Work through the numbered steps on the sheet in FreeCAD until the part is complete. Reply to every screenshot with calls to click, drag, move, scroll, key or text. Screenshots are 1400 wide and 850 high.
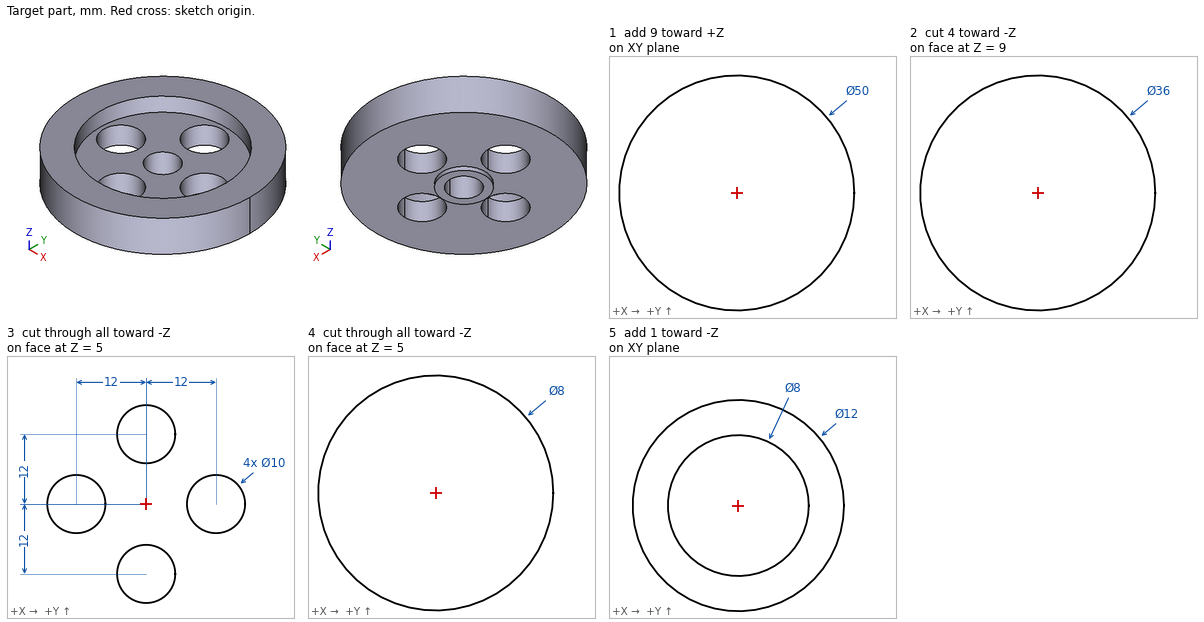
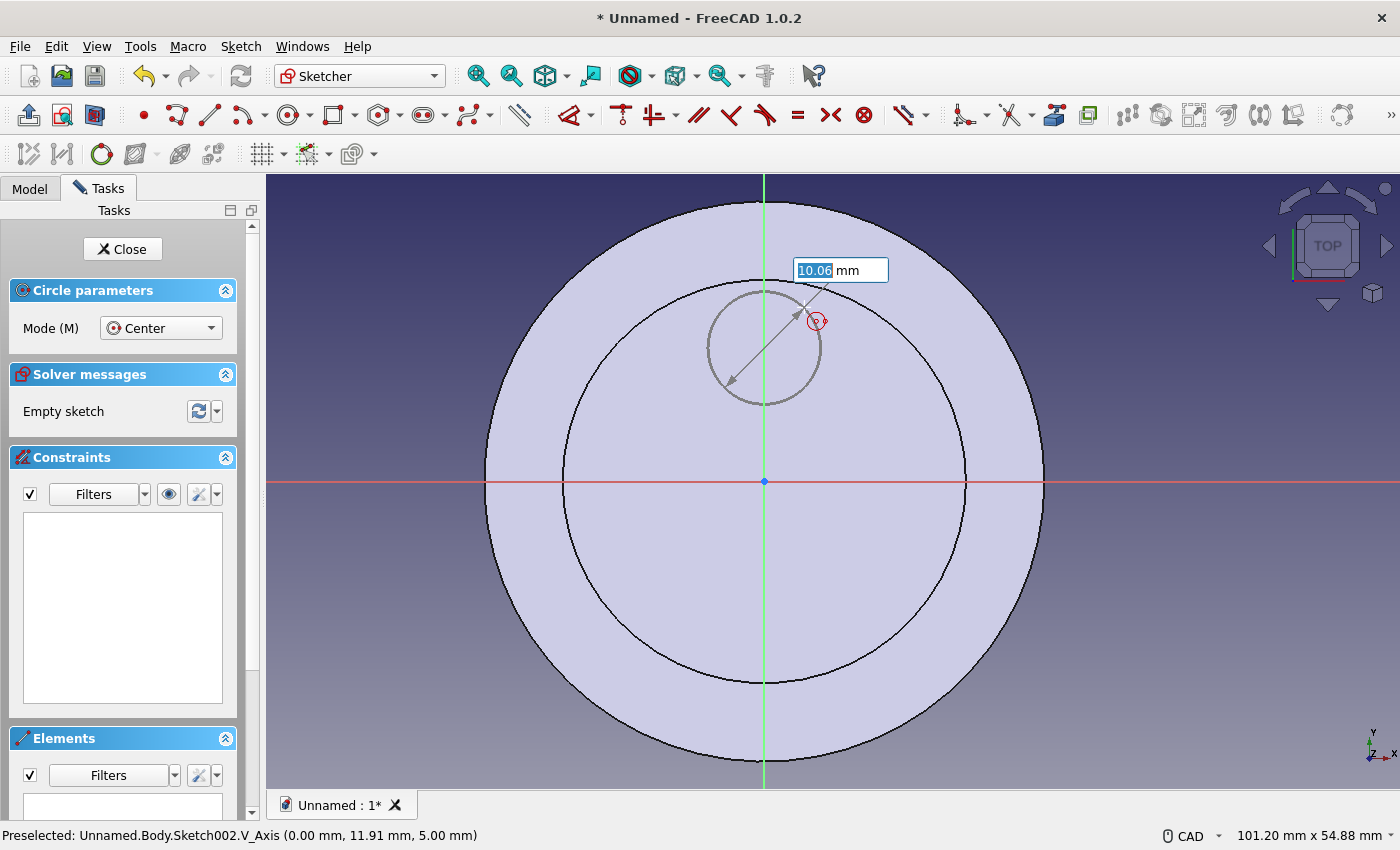
text(10)
key(Return)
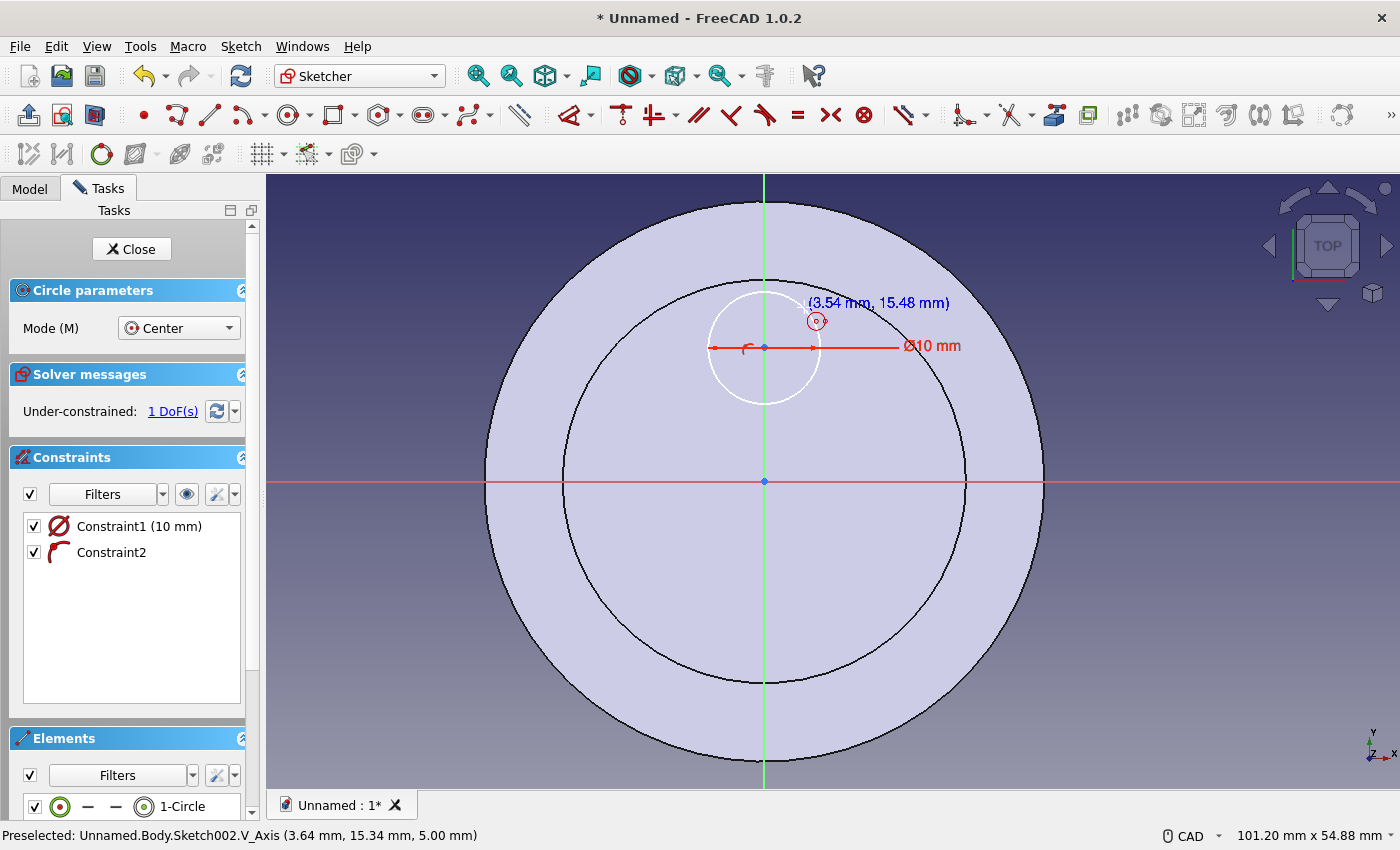
click(899, 482)
move(938, 442)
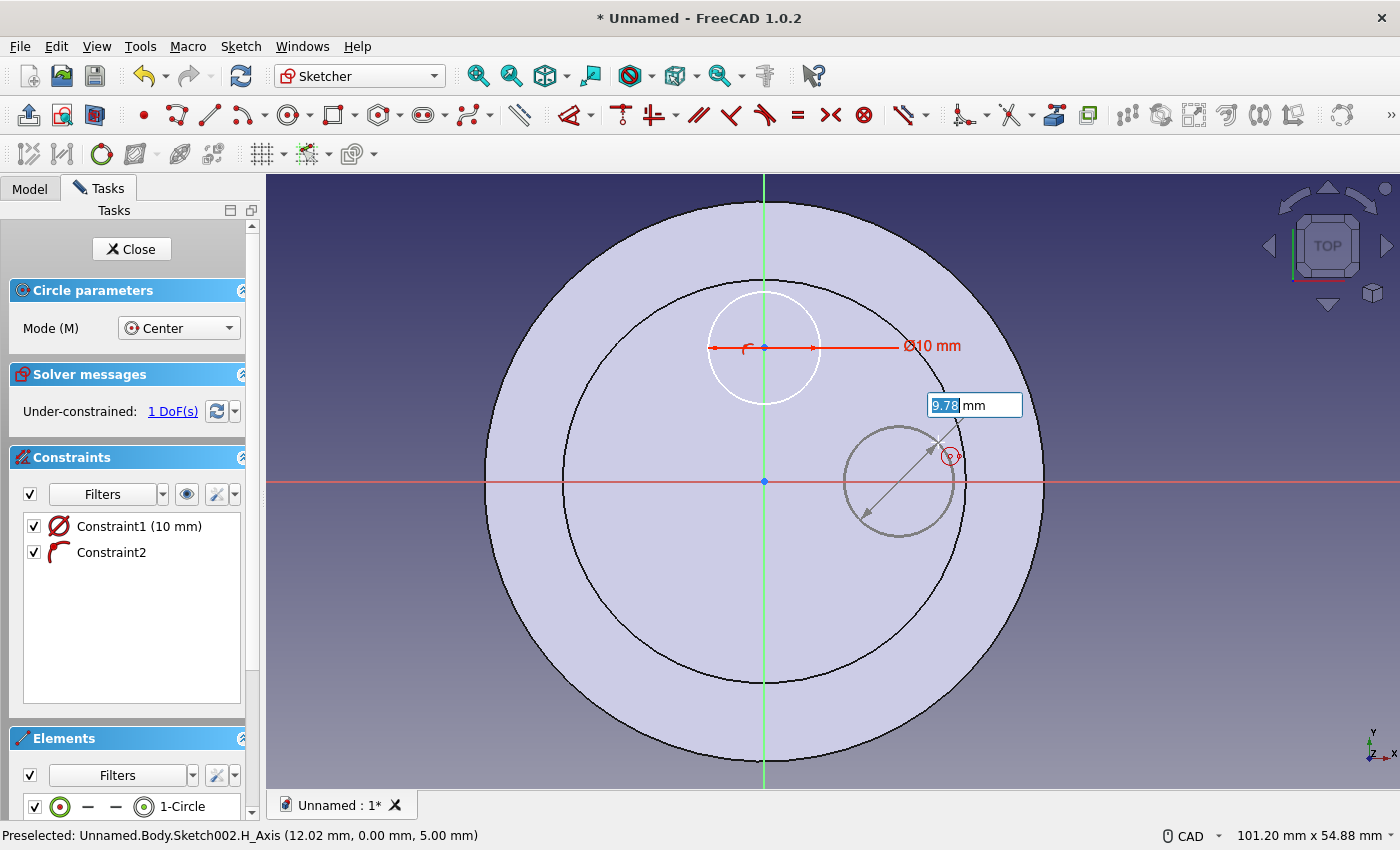
text(10)
key(Return)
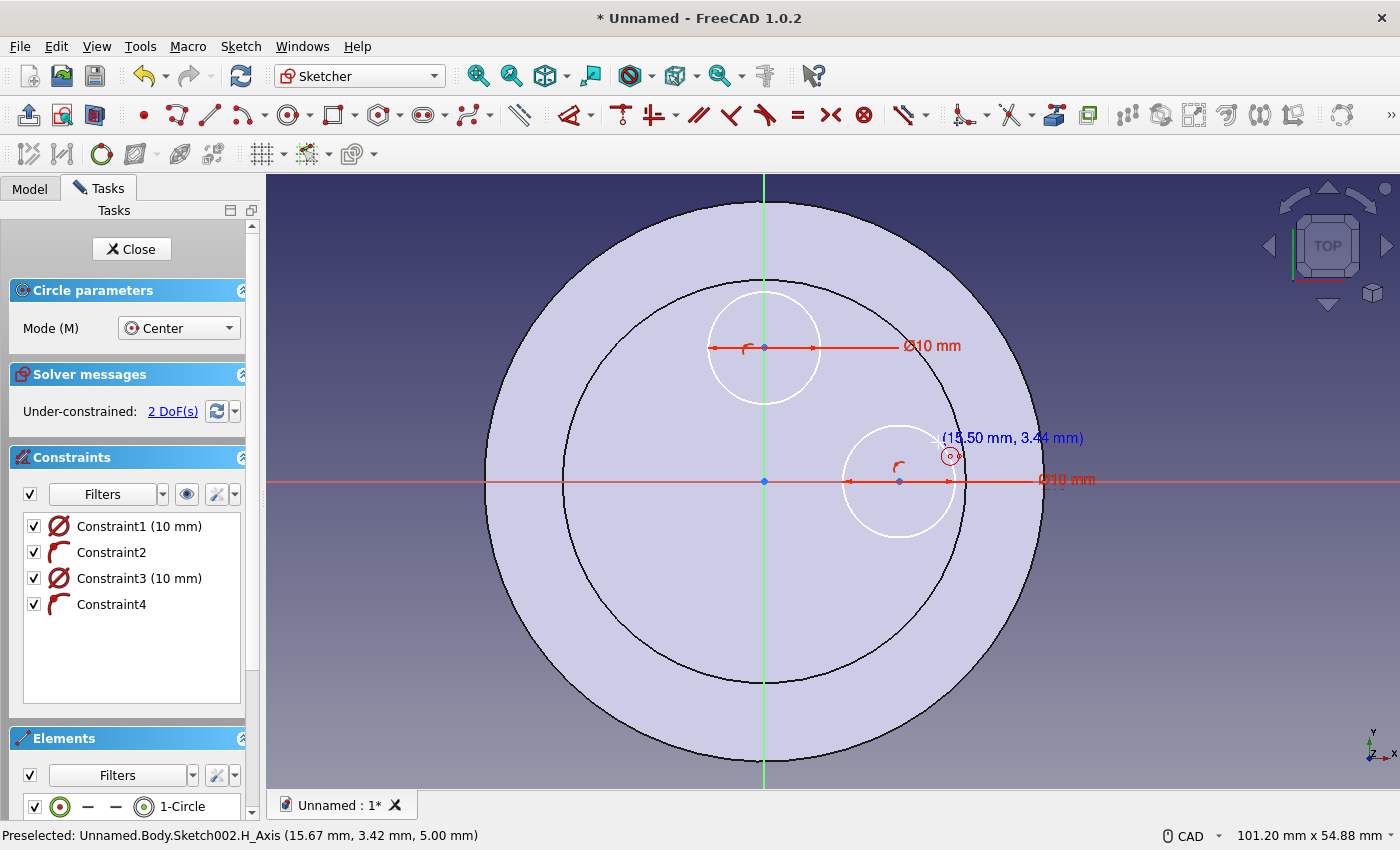
click(764, 616)
move(804, 576)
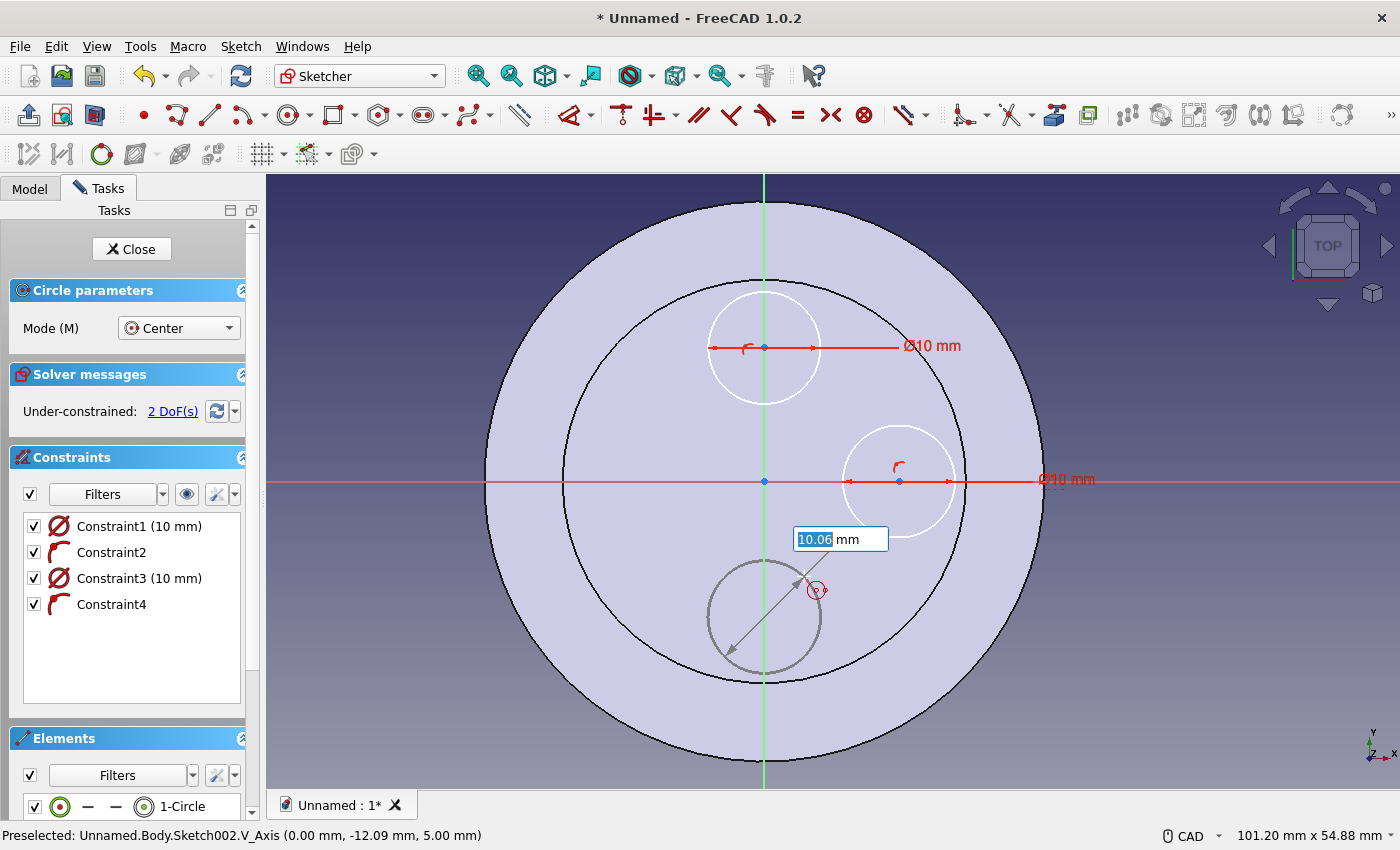
text(10)
key(Return)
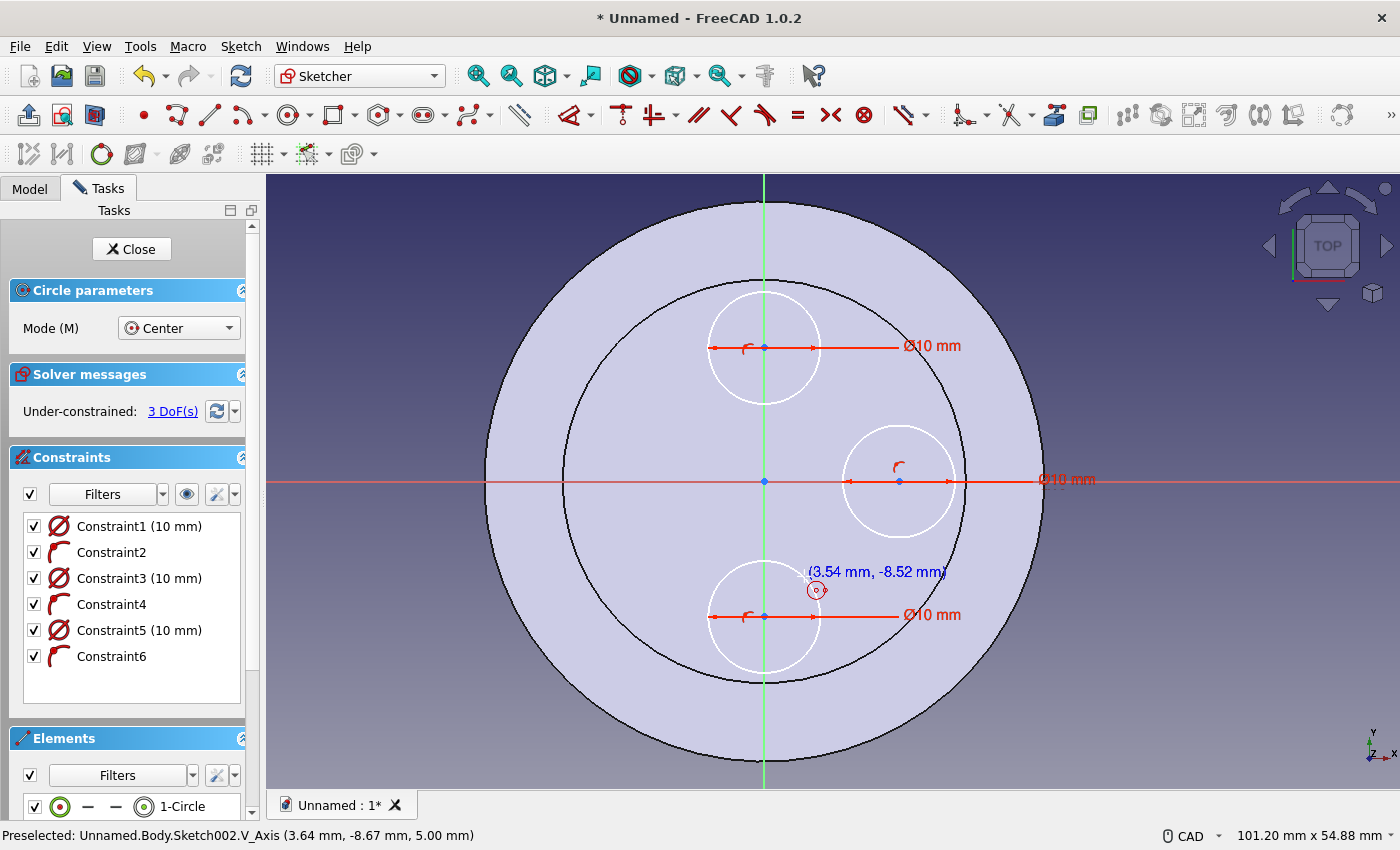
click(630, 482)
move(669, 442)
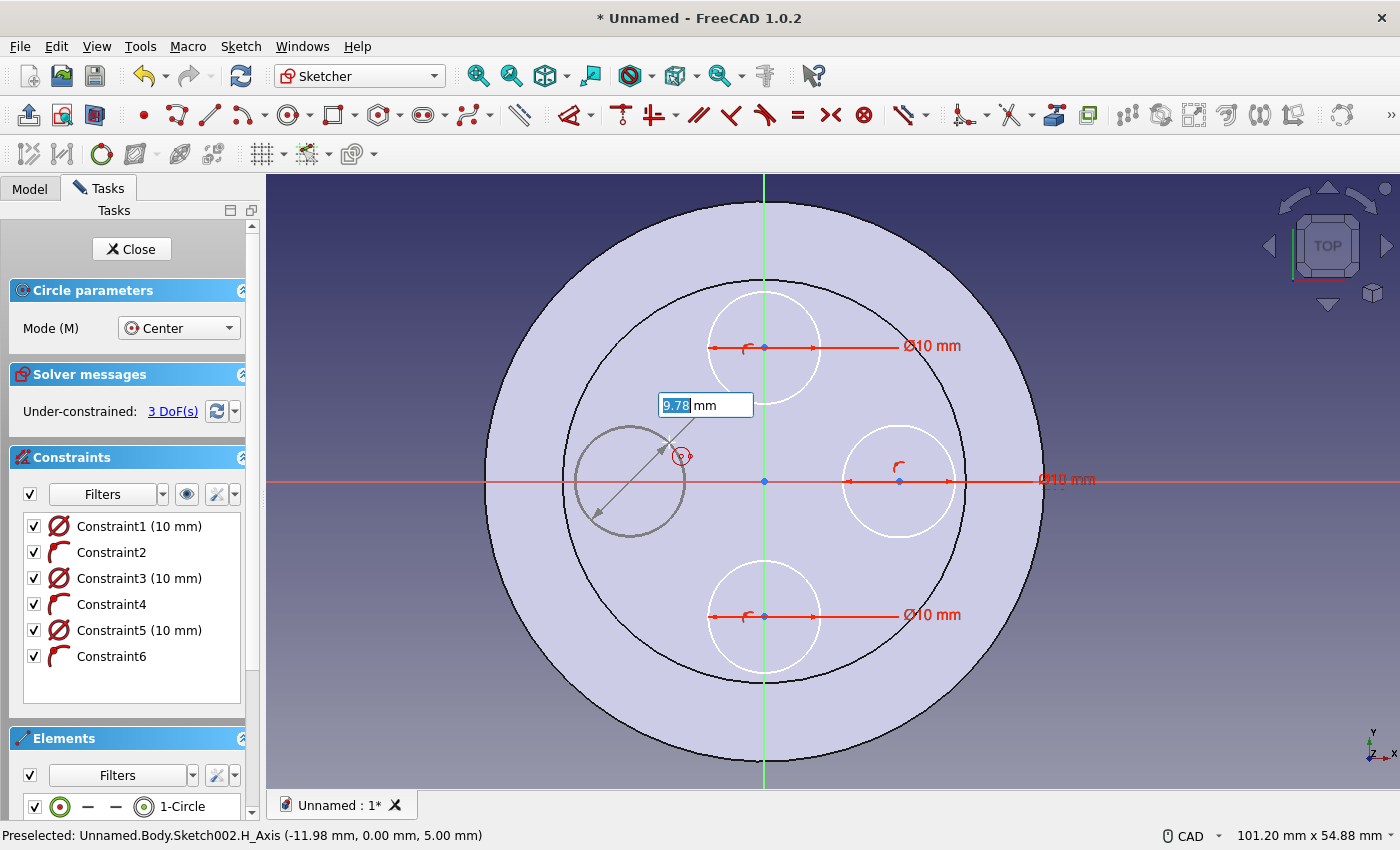
text(10)
key(Return)
key(Escape)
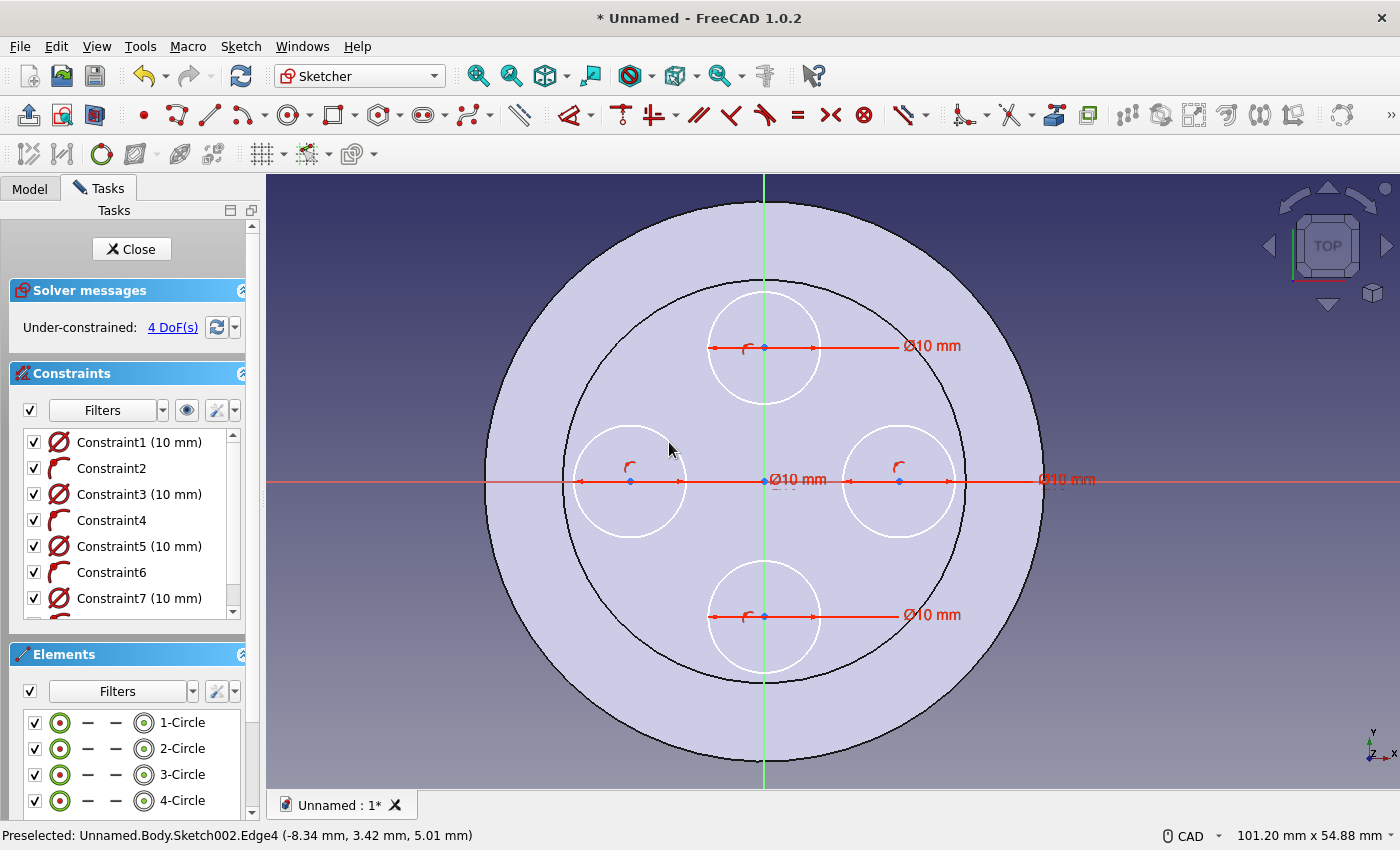
click(568, 116)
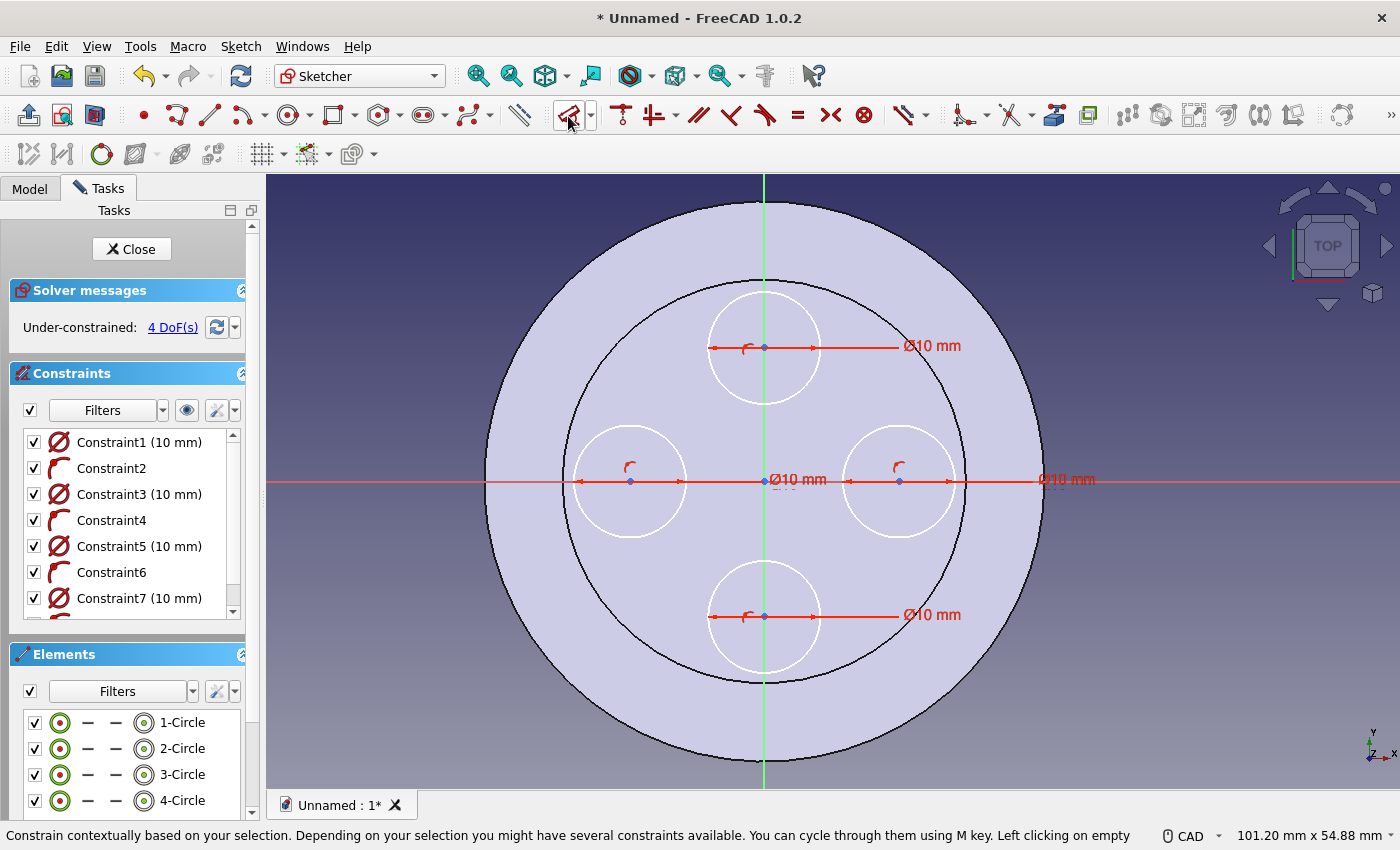
click(764, 348)
click(798, 415)